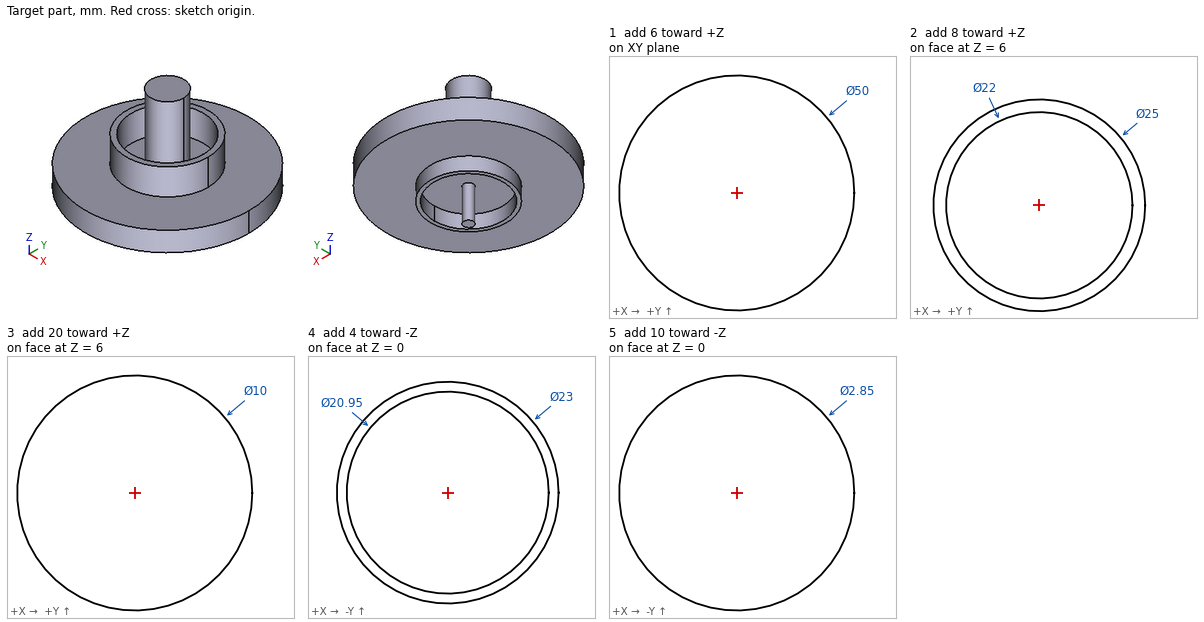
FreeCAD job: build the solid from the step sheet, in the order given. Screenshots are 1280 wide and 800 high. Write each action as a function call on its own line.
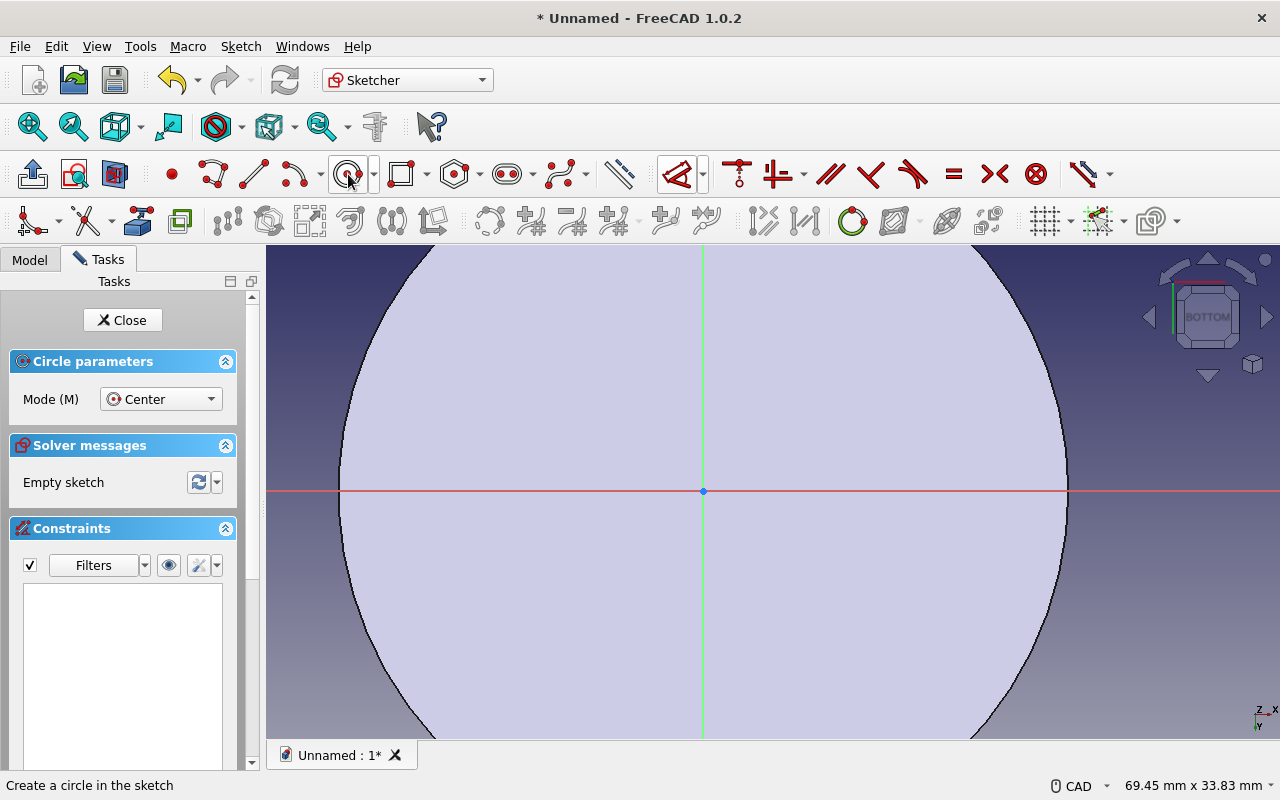
click(703, 491)
click(822, 373)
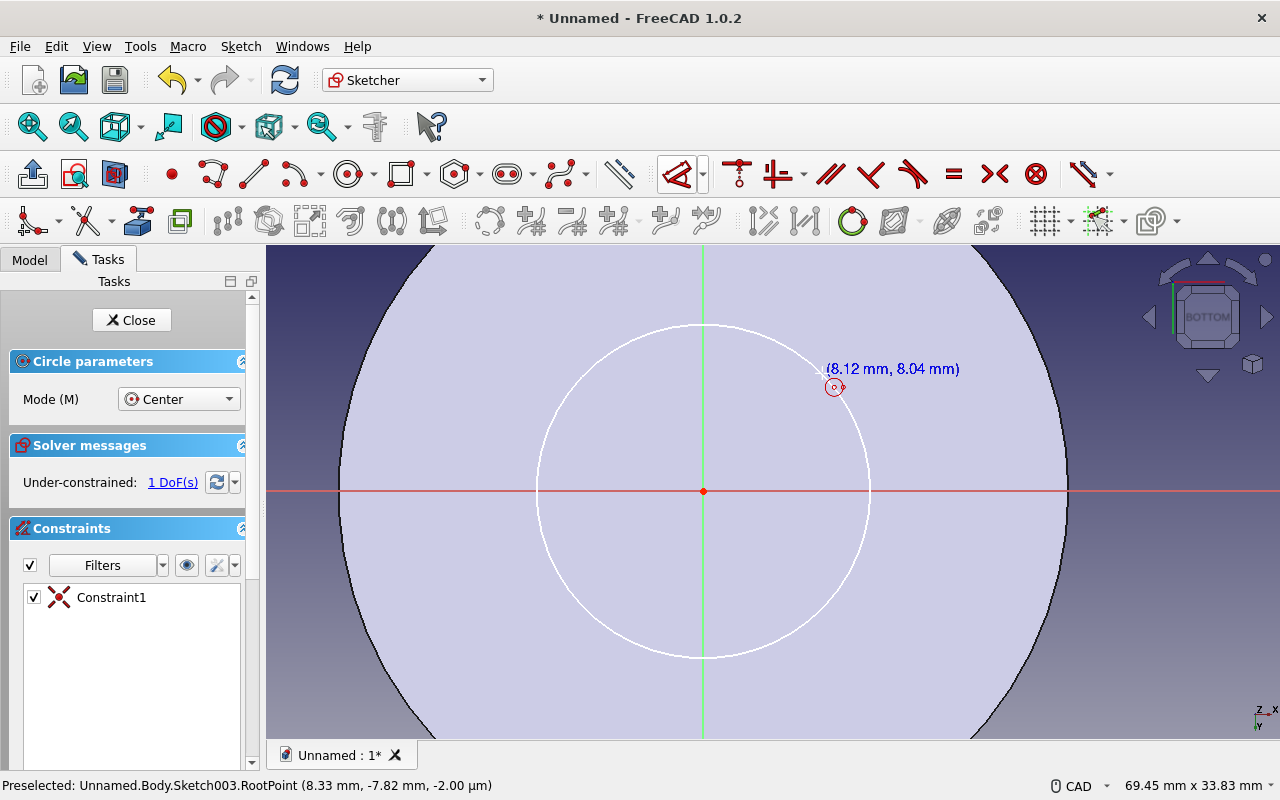
click(703, 491)
click(812, 383)
key(Escape)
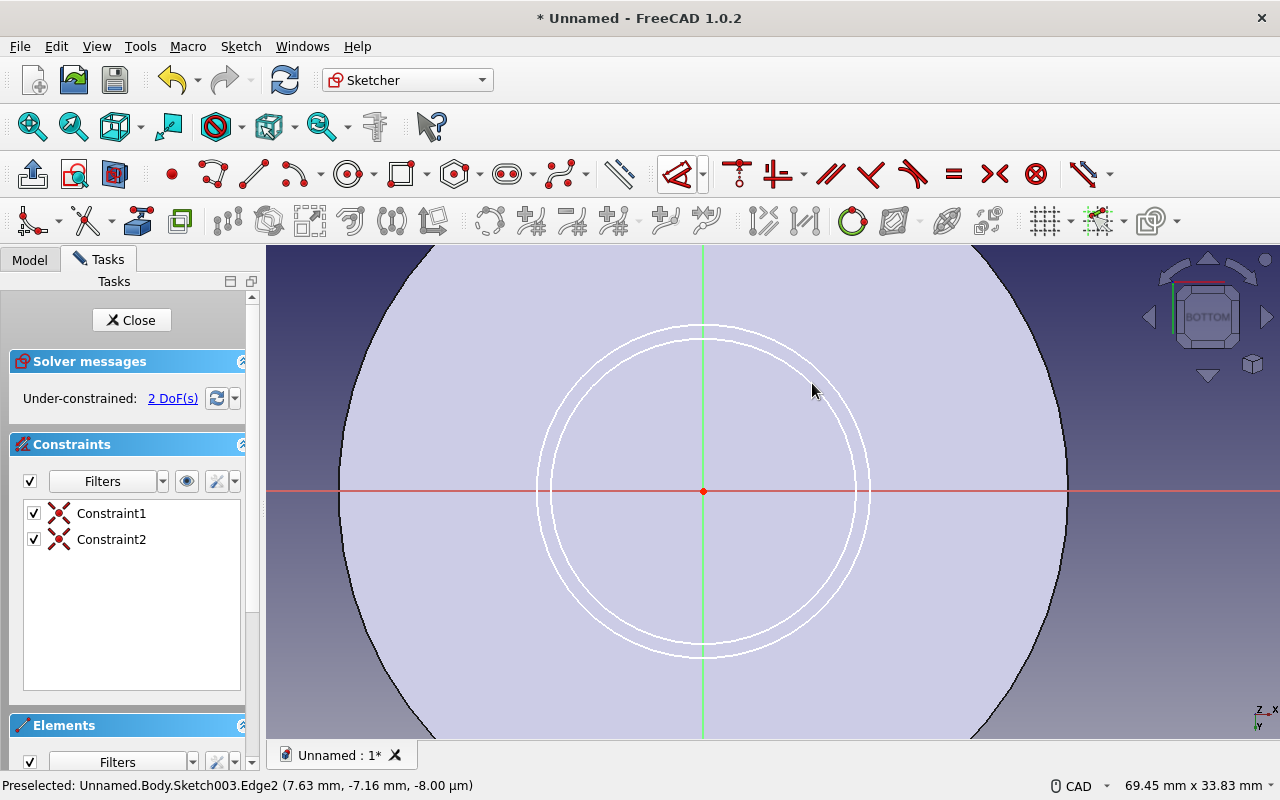
click(821, 373)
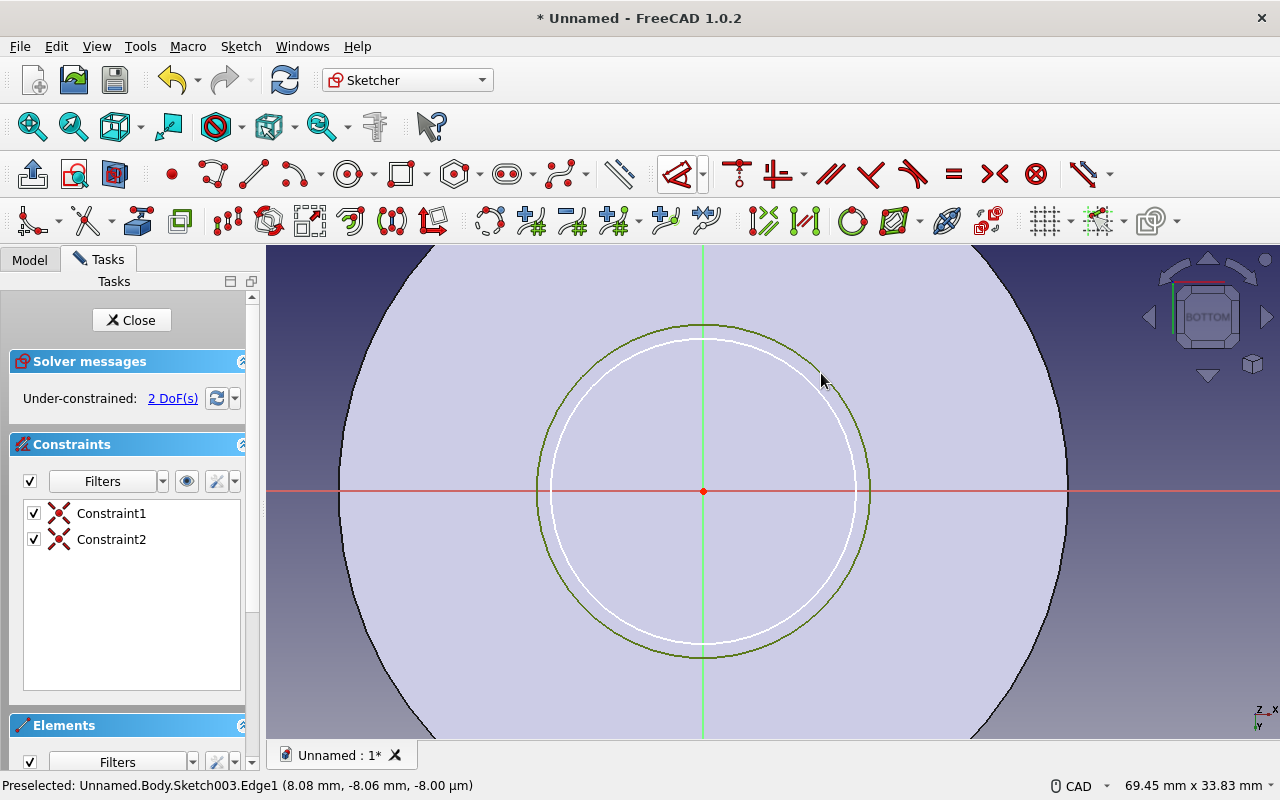
click(702, 174)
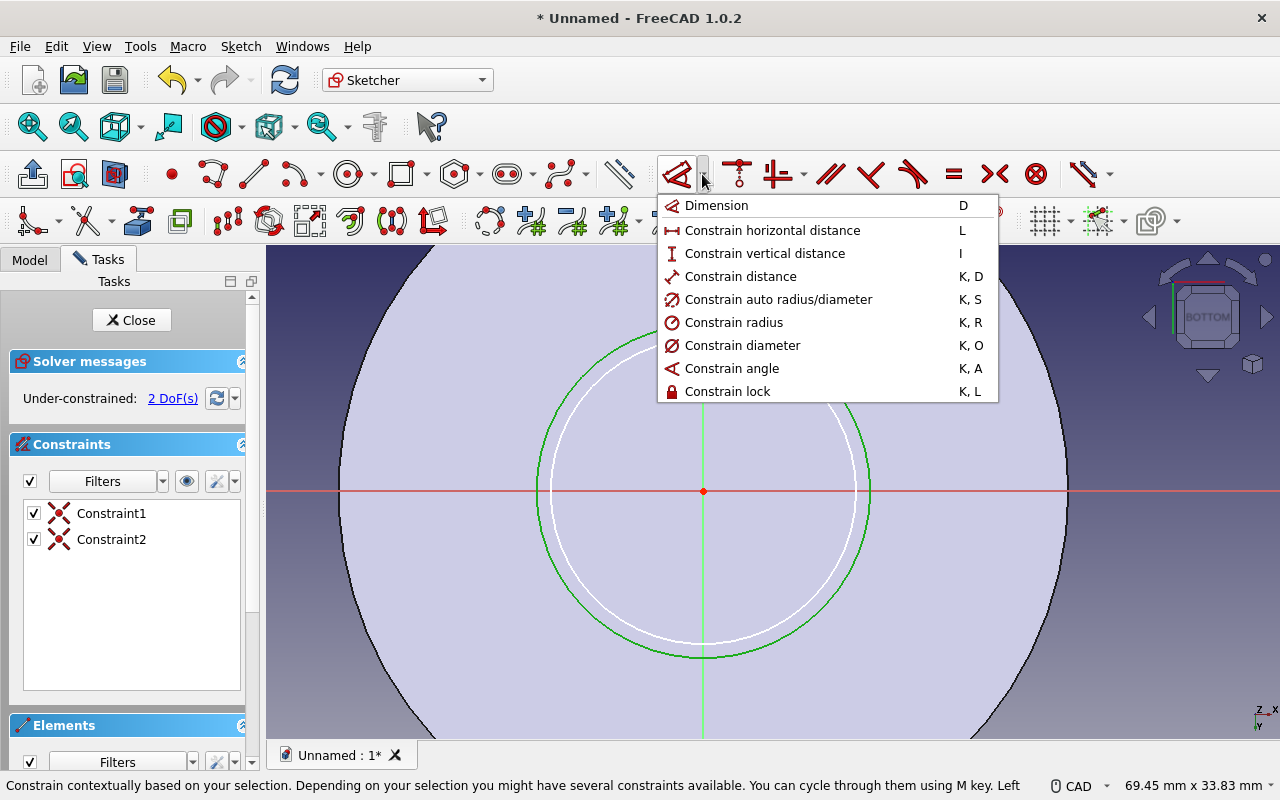
click(828, 346)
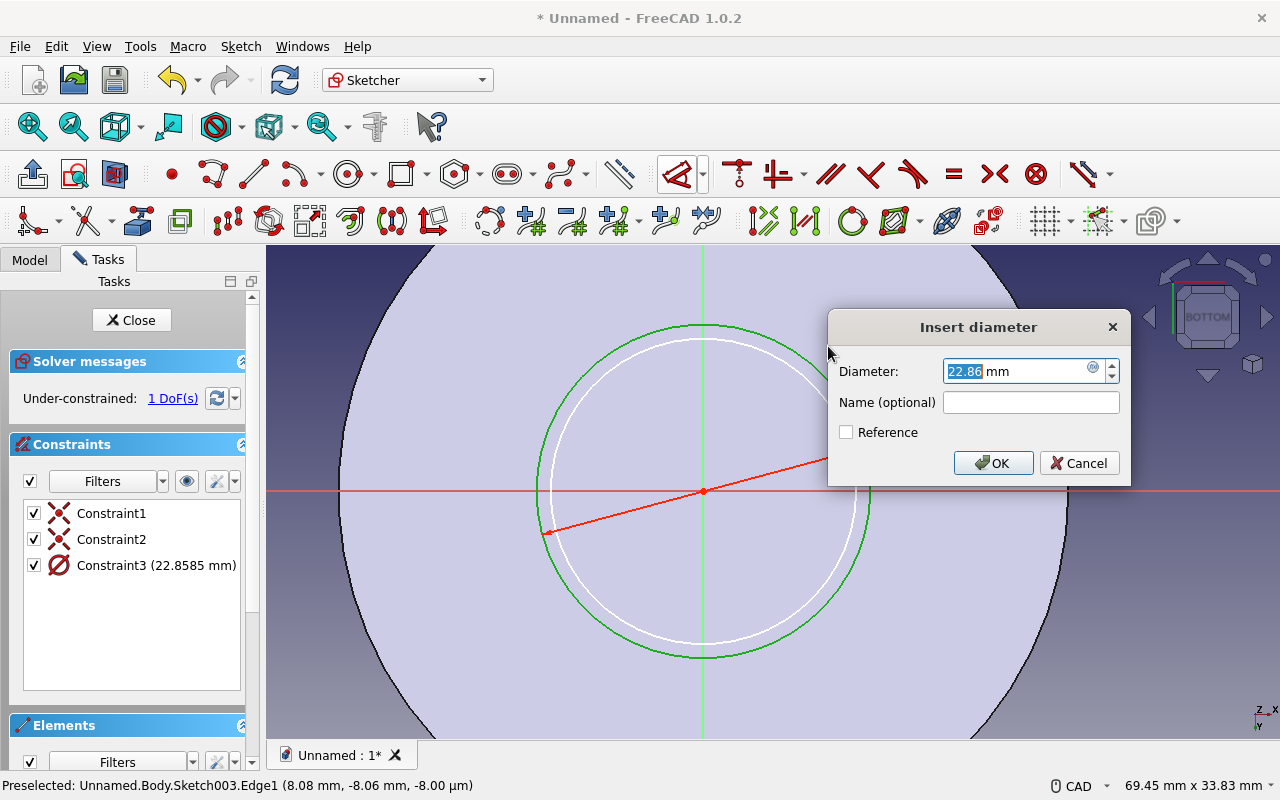
text(23)
key(Return)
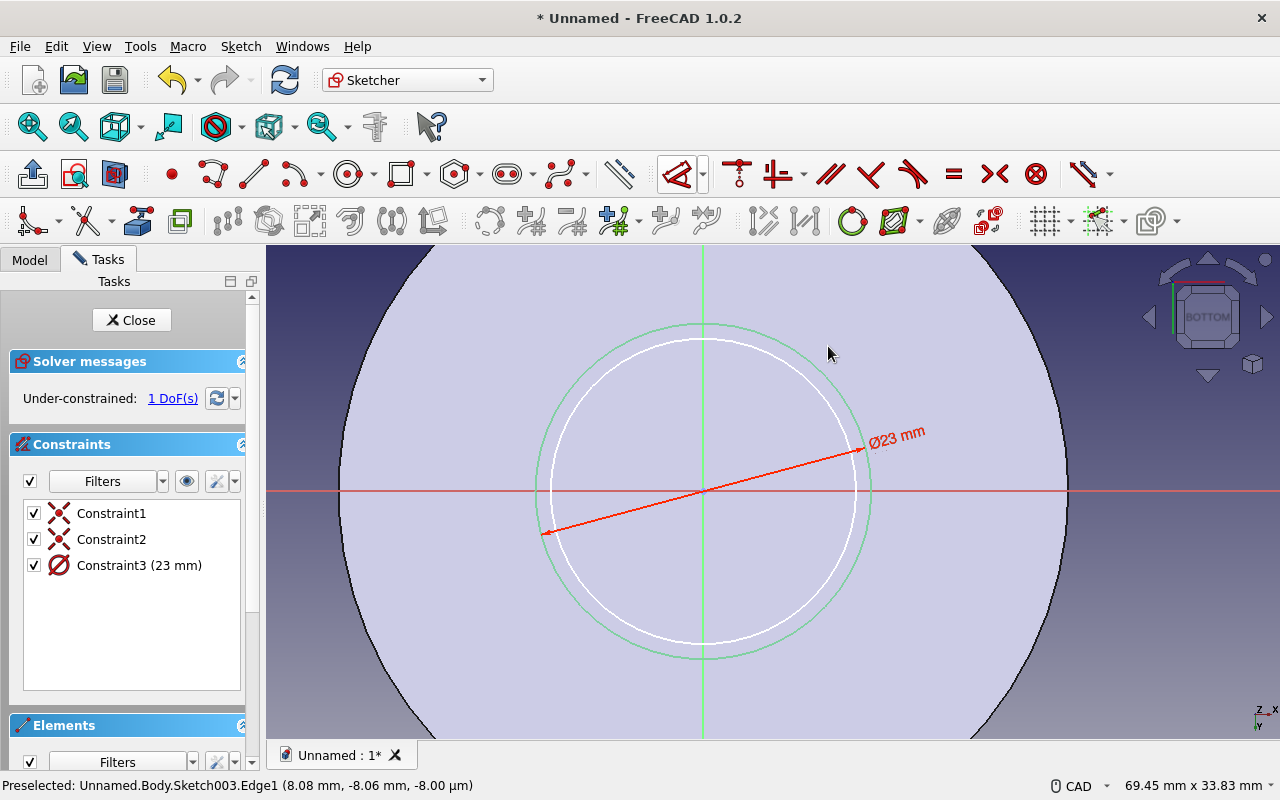
click(811, 383)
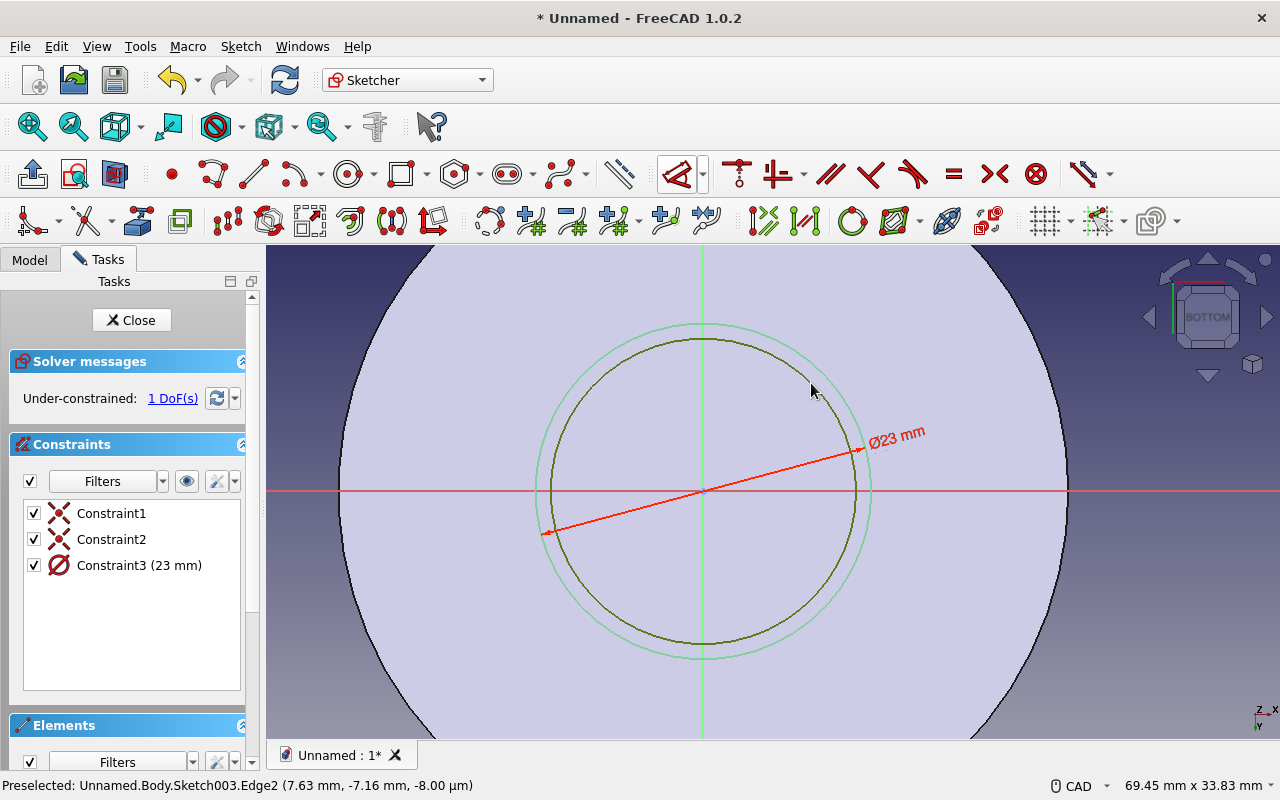
click(702, 174)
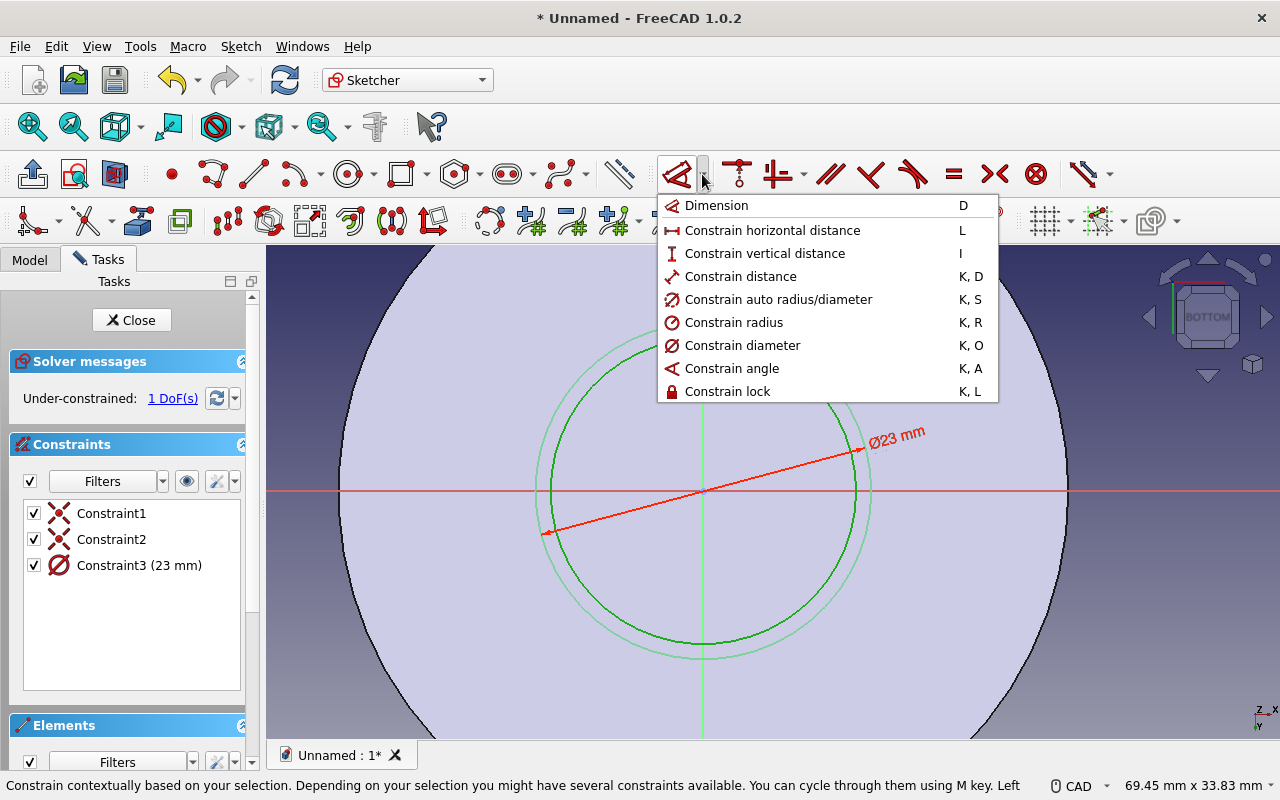
click(828, 346)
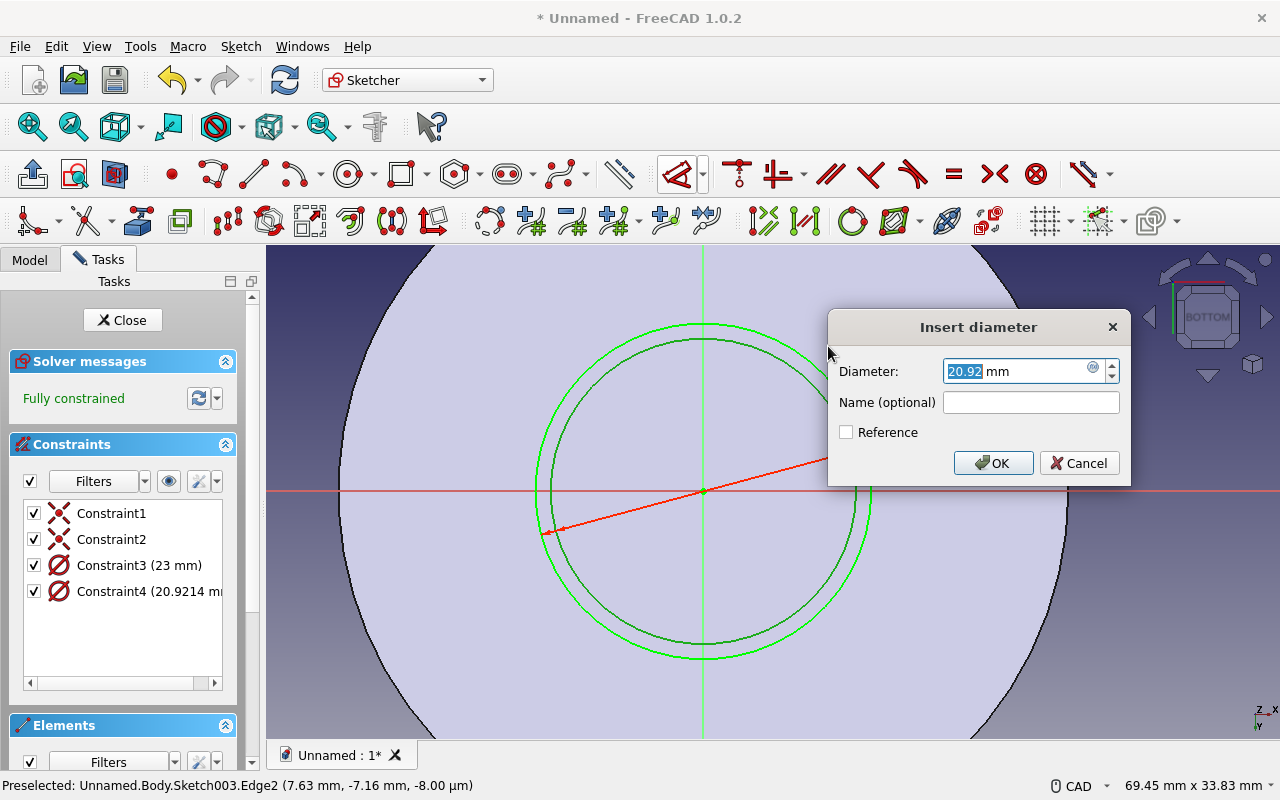
text(20.95)
key(Return)